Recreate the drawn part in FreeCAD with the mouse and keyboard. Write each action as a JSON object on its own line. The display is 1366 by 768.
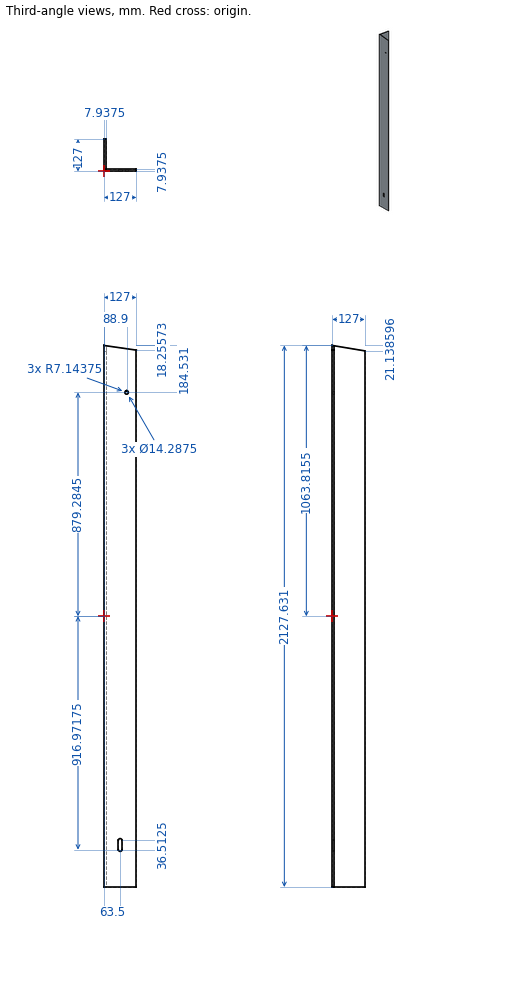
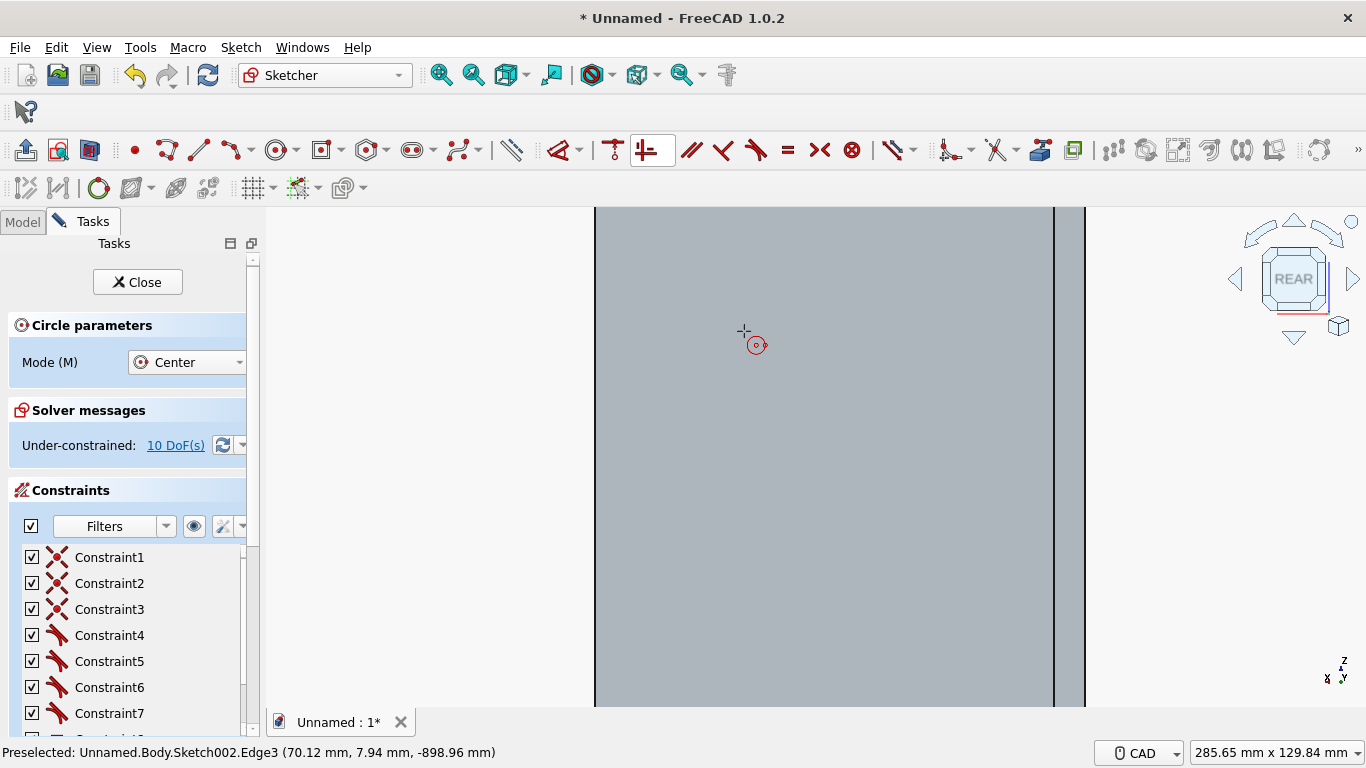
{"action": "scroll", "coordinate": [743, 301], "scroll_direction": "down", "scroll_amount": 15}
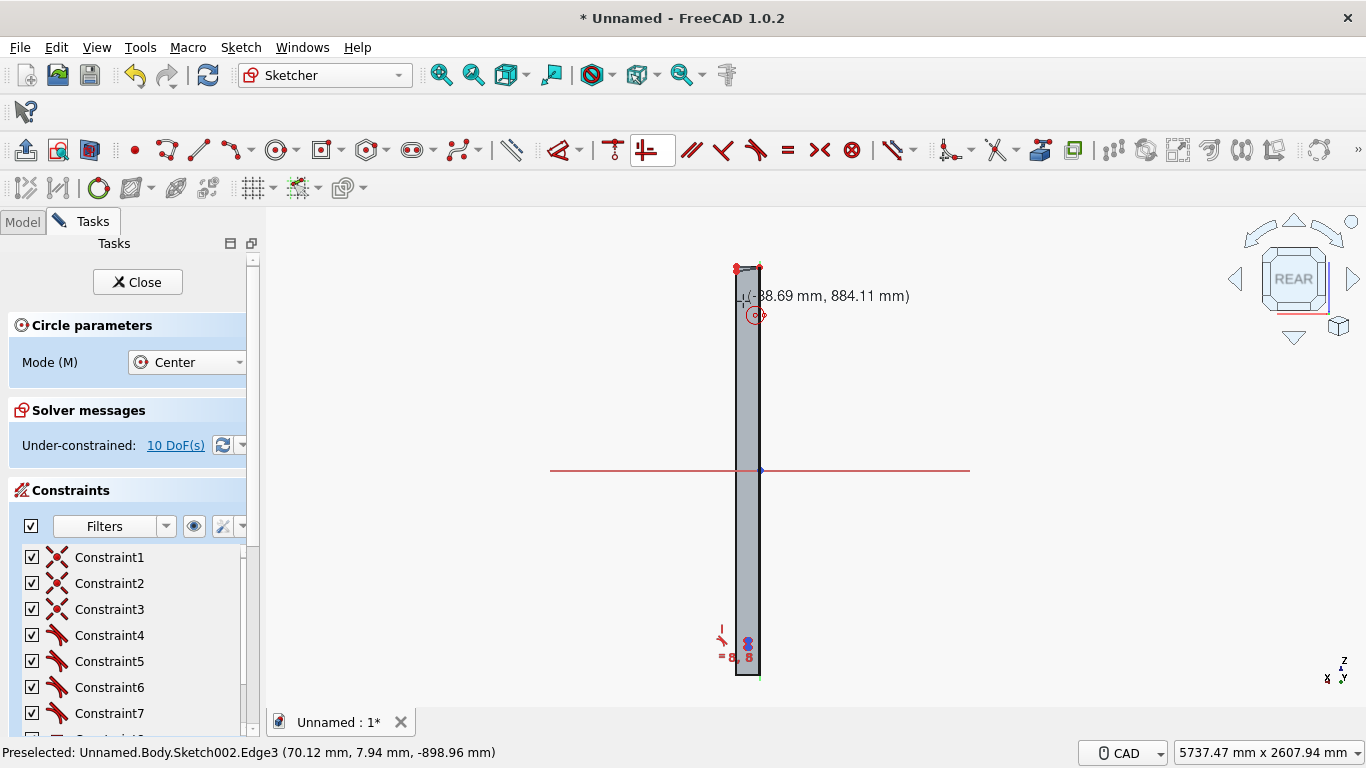
{"action": "left_click", "coordinate": [743, 302]}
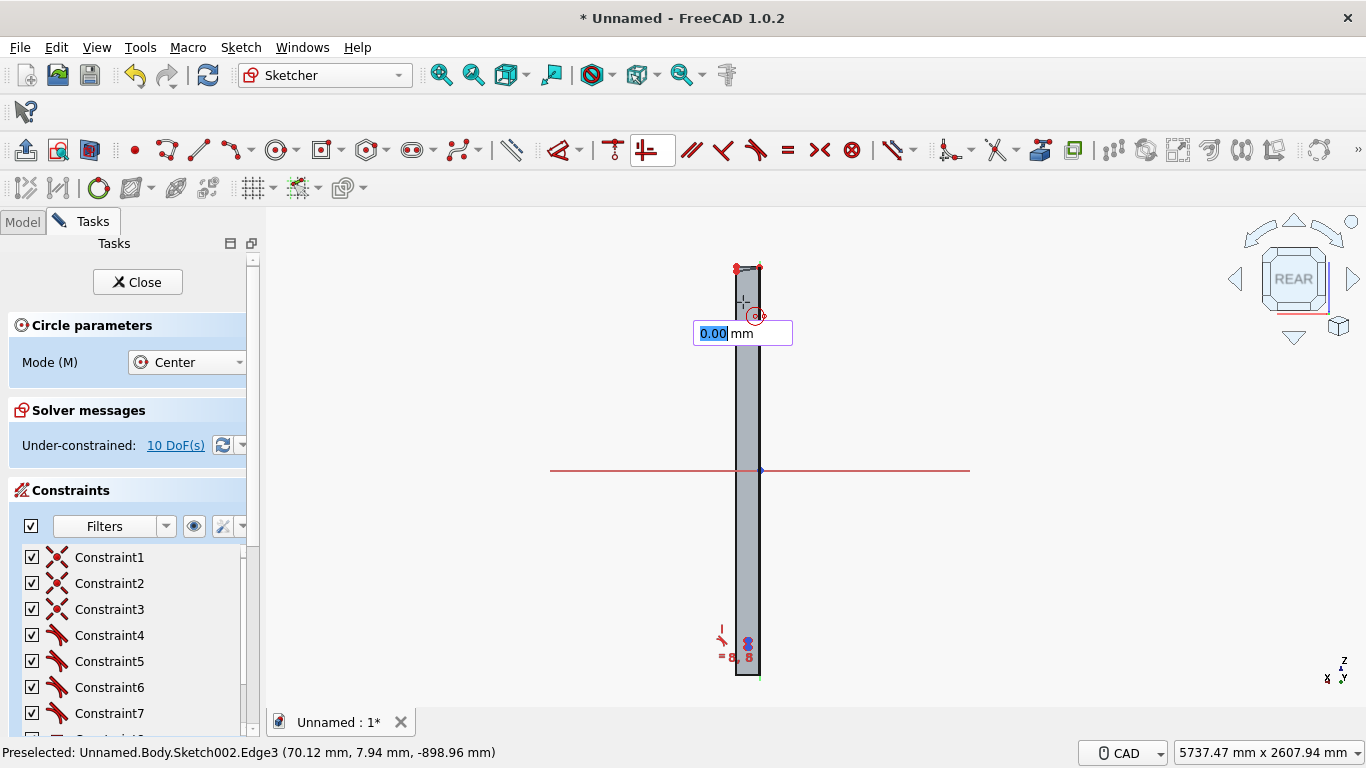
{"action": "scroll", "coordinate": [744, 301], "scroll_direction": "up", "scroll_amount": 13}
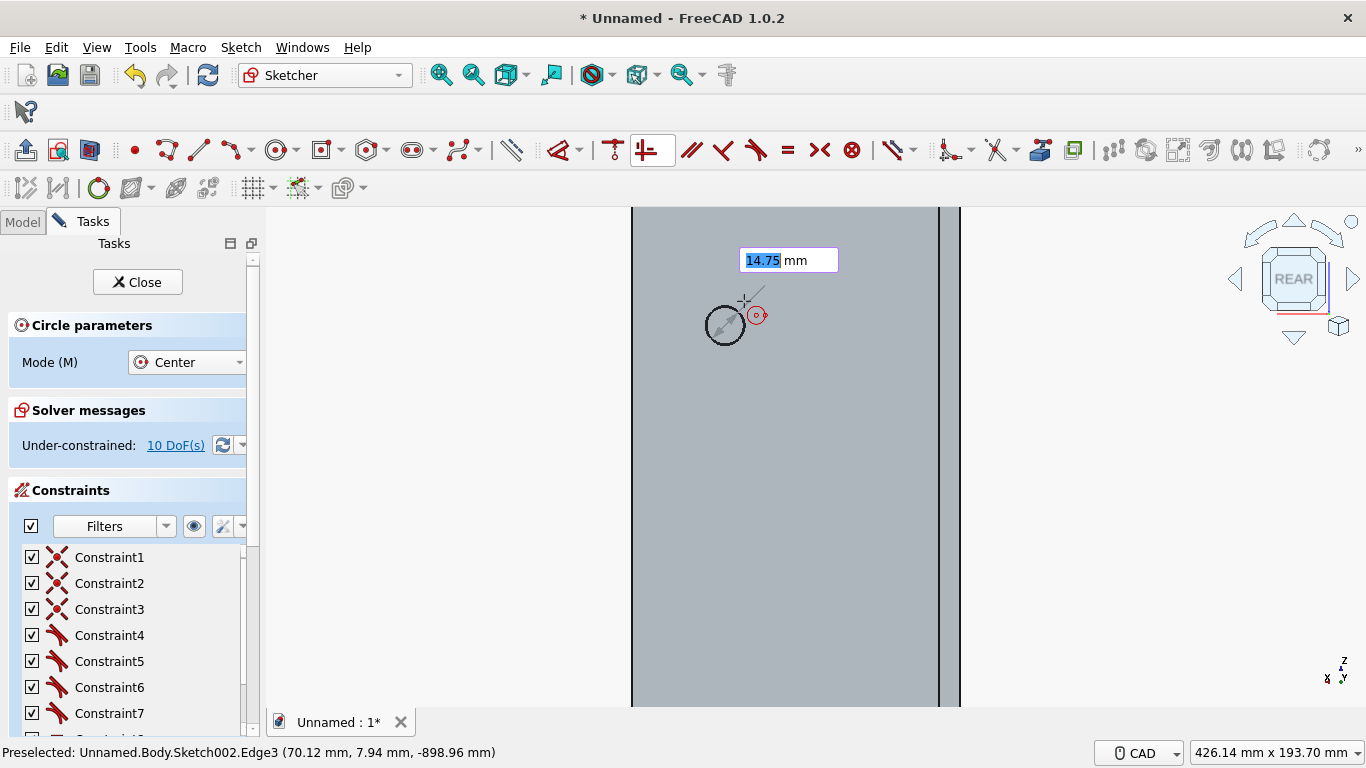
{"action": "left_click", "coordinate": [743, 301]}
{"action": "key", "text": "Escape"}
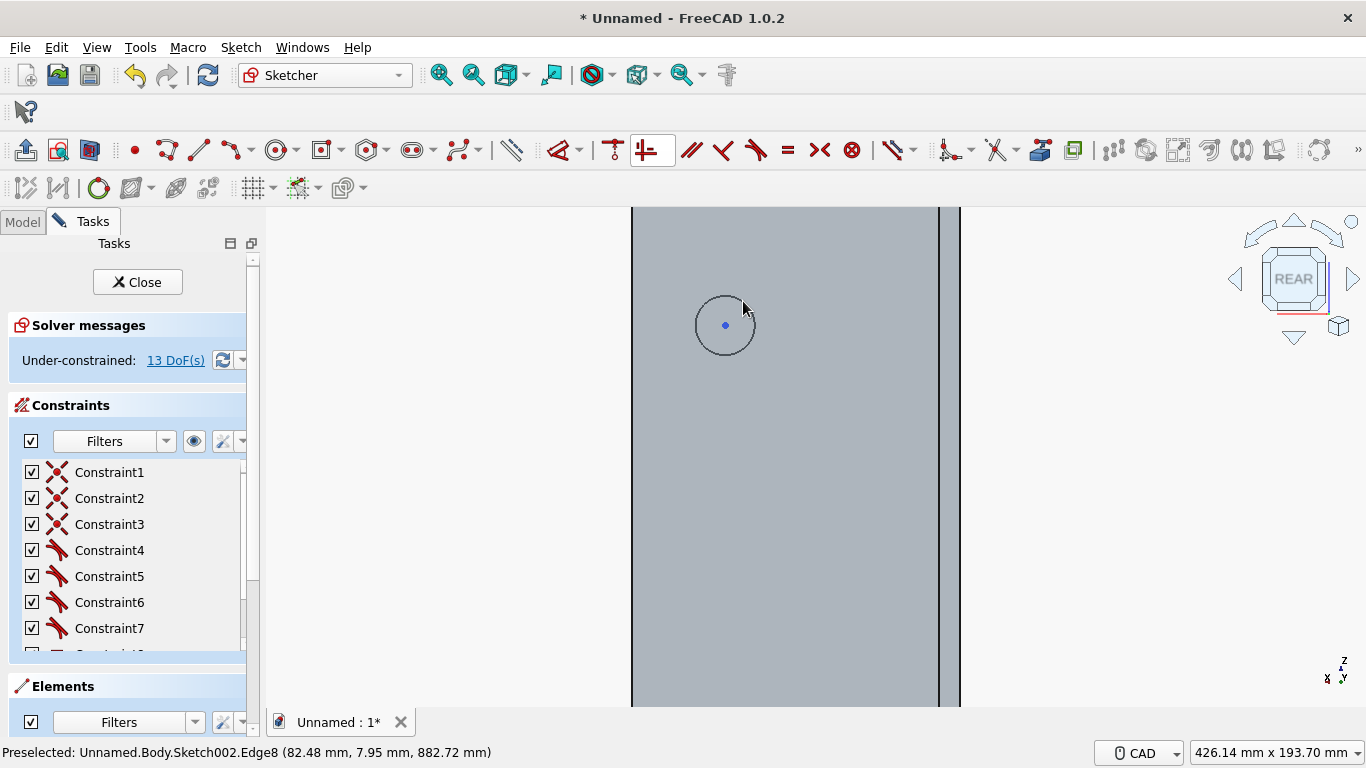
{"action": "scroll", "coordinate": [744, 331], "scroll_direction": "down", "scroll_amount": 14}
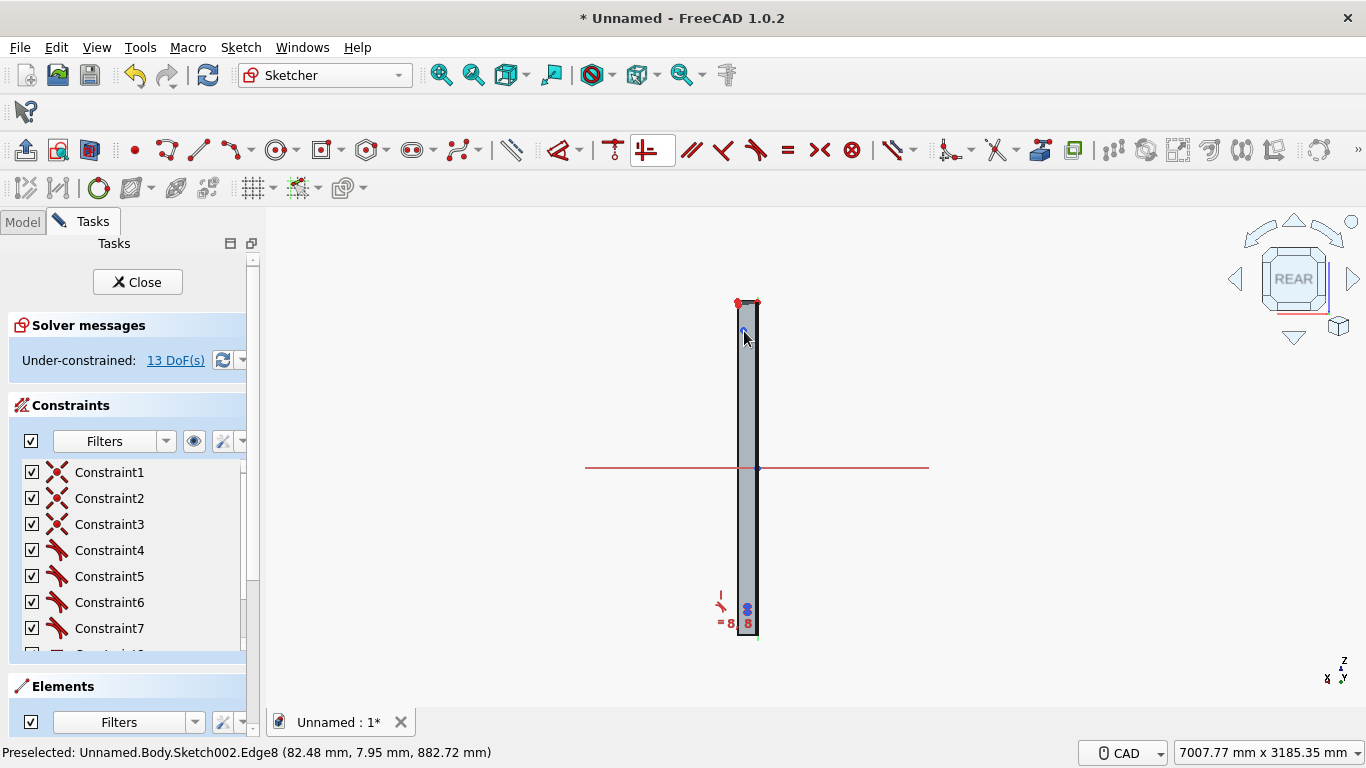
{"action": "scroll", "coordinate": [751, 302], "scroll_direction": "up", "scroll_amount": 13}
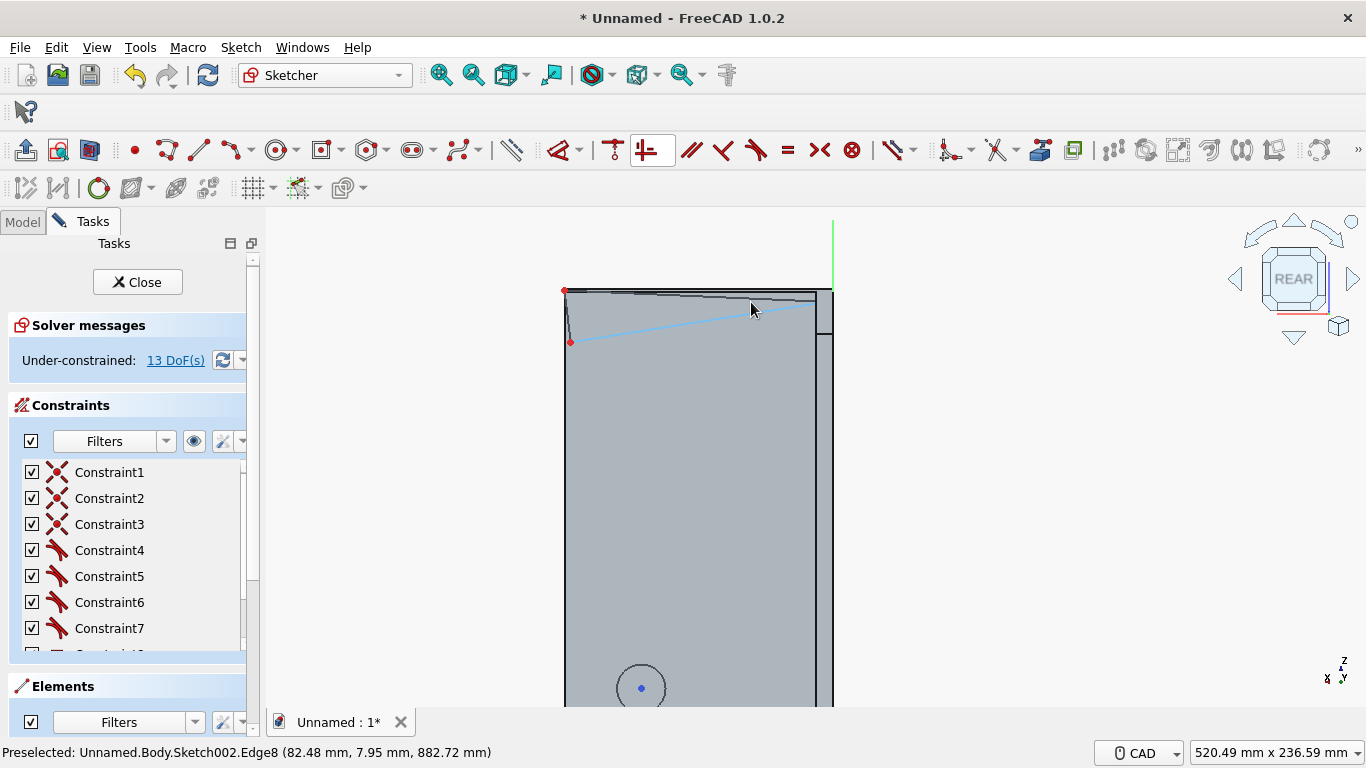
{"action": "left_click", "coordinate": [748, 298]}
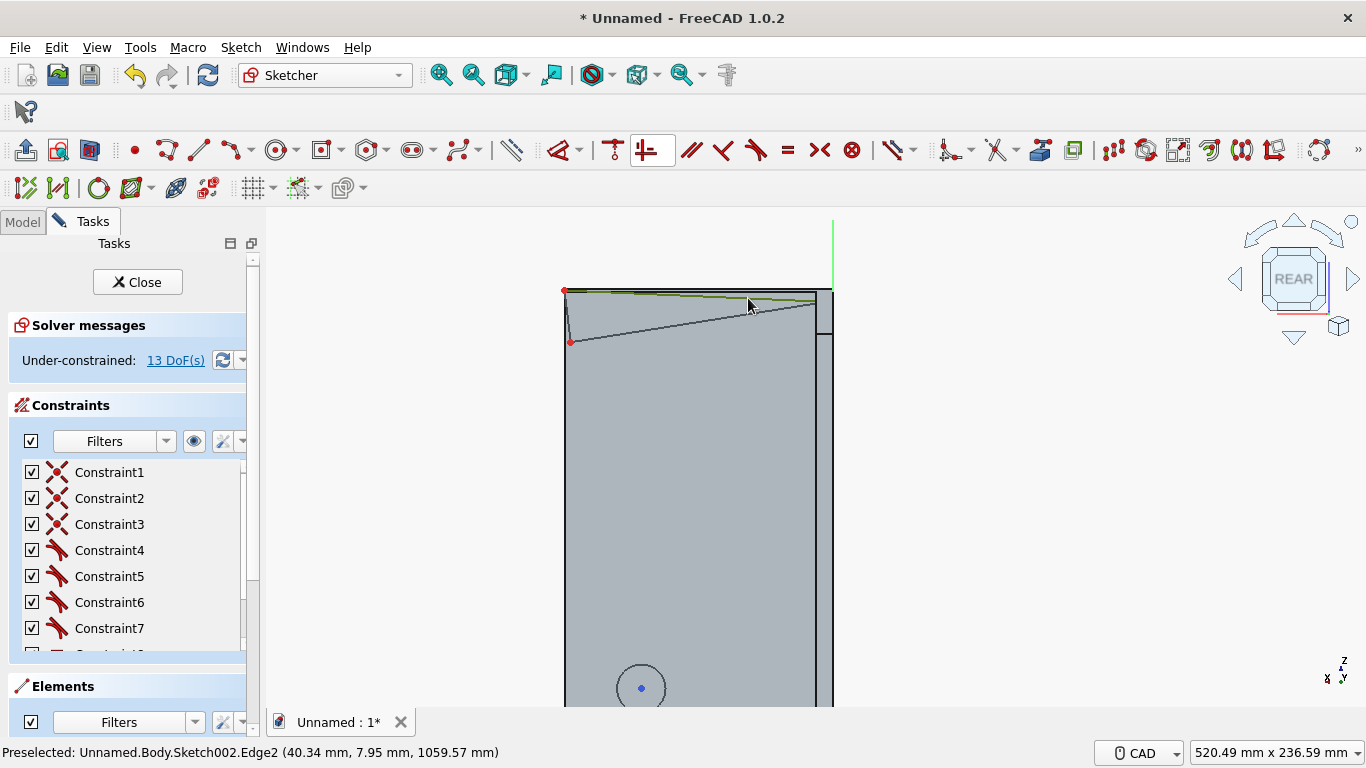
{"action": "left_click", "coordinate": [670, 150]}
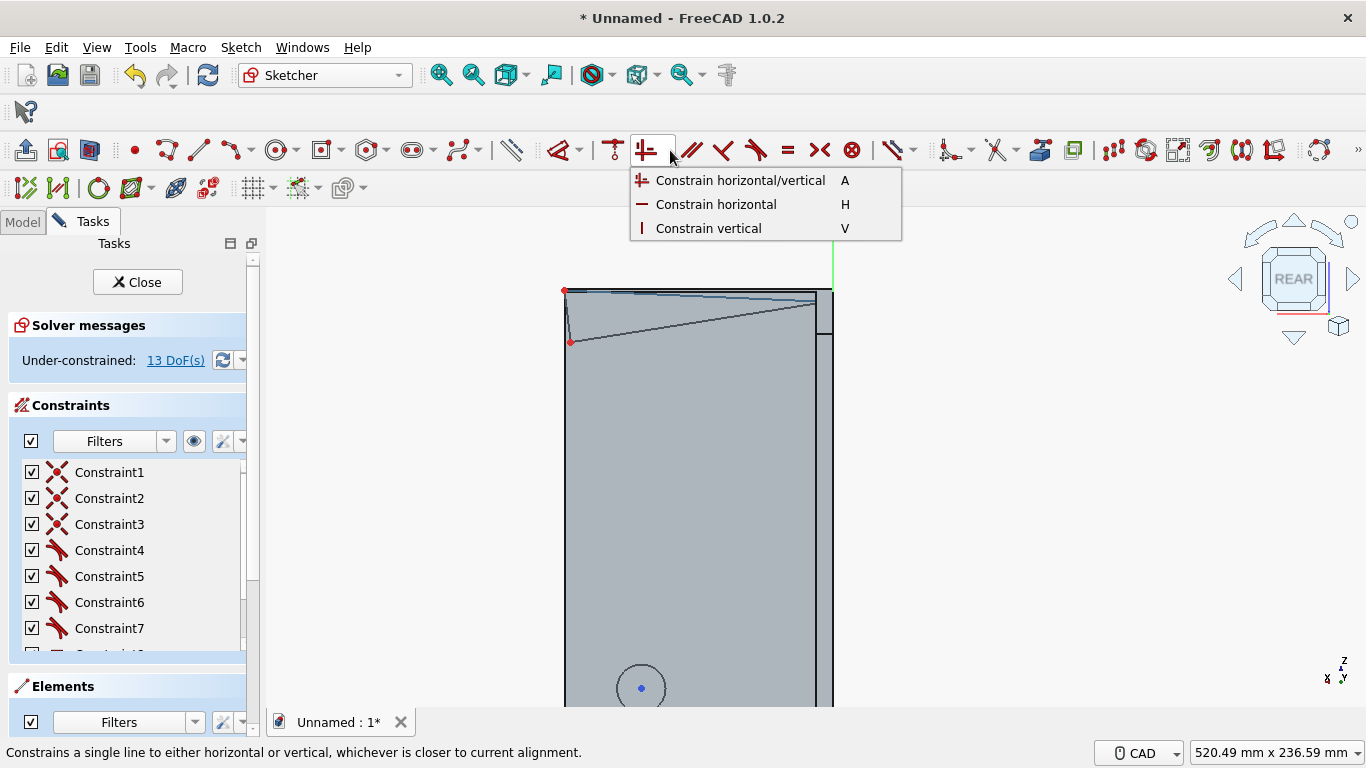
{"action": "left_click", "coordinate": [766, 204]}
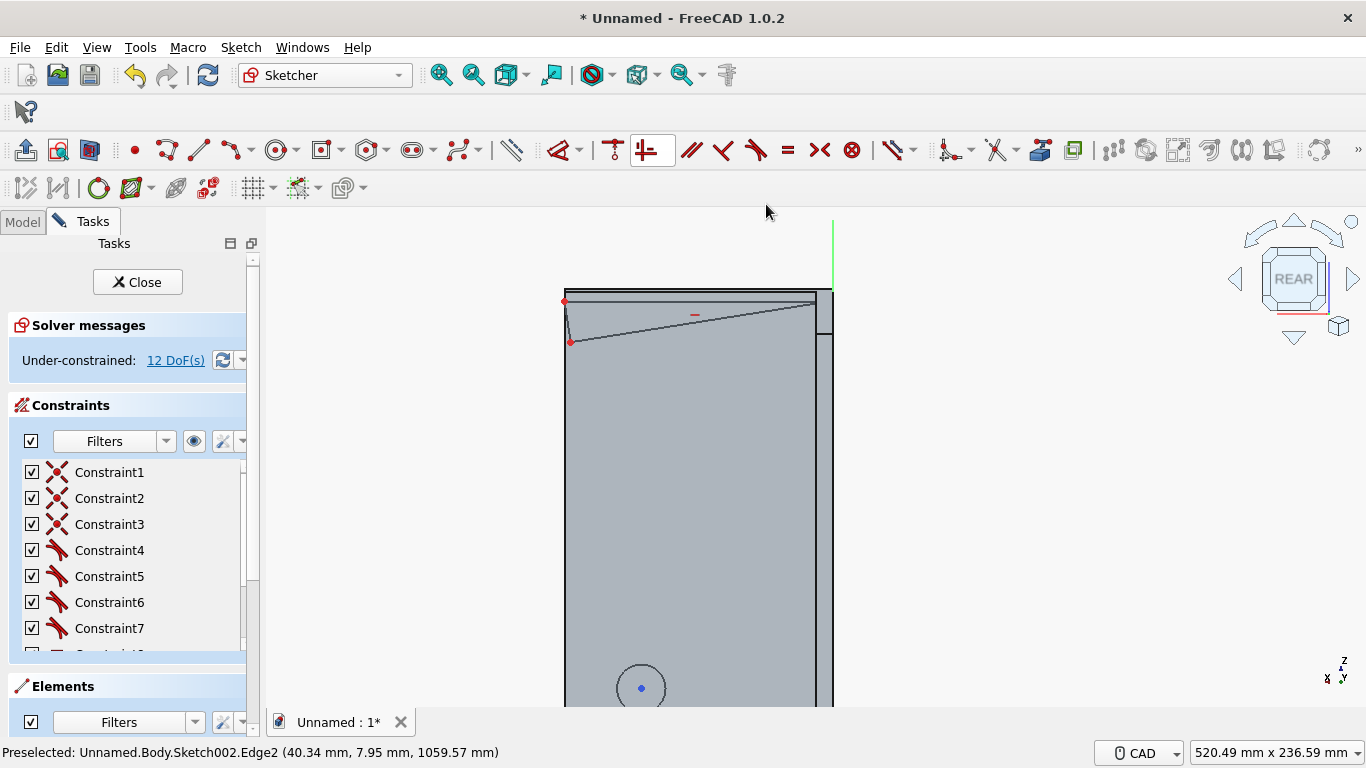
{"action": "left_click", "coordinate": [566, 314]}